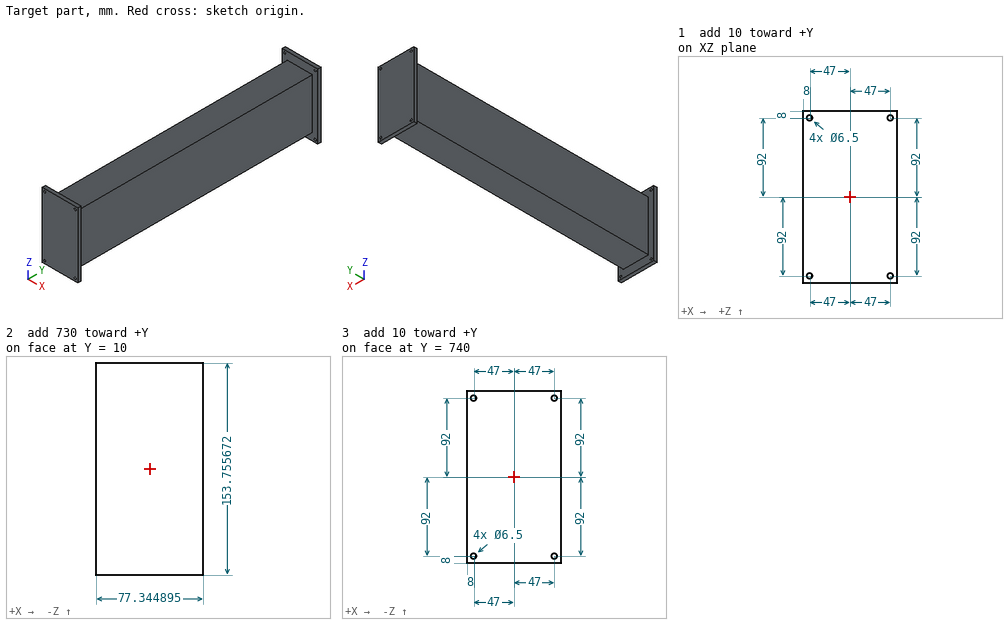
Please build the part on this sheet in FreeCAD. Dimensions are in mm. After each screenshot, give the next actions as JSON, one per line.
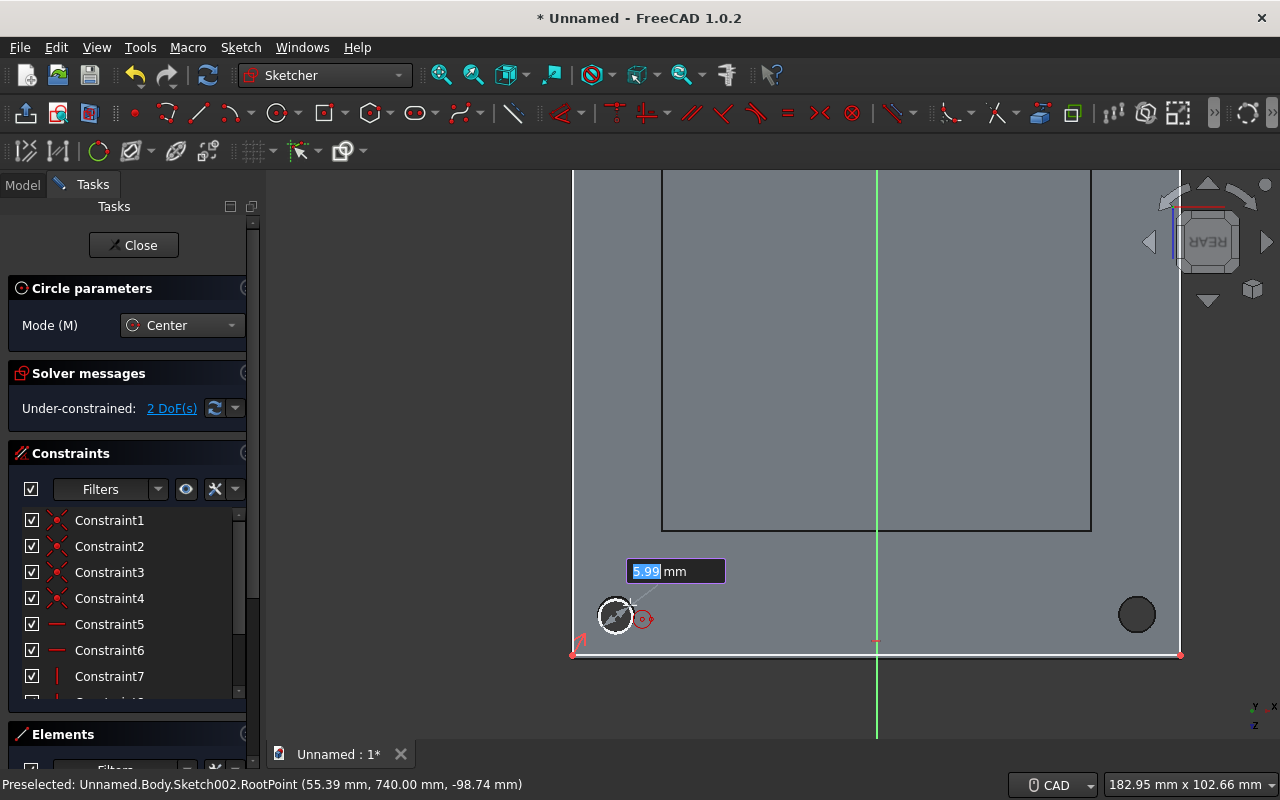
{"action": "left_click", "coordinate": [629, 602]}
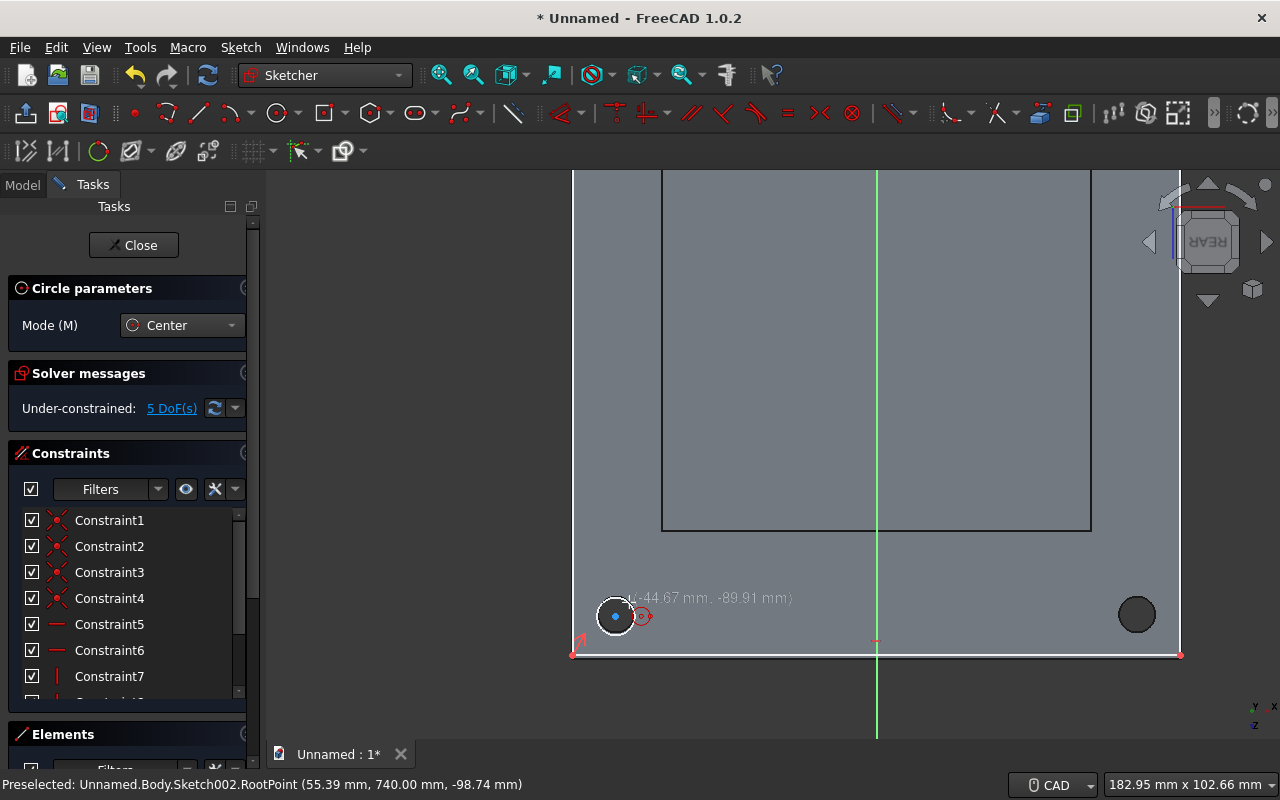
{"action": "scroll", "coordinate": [630, 605], "scroll_direction": "down", "scroll_amount": 6}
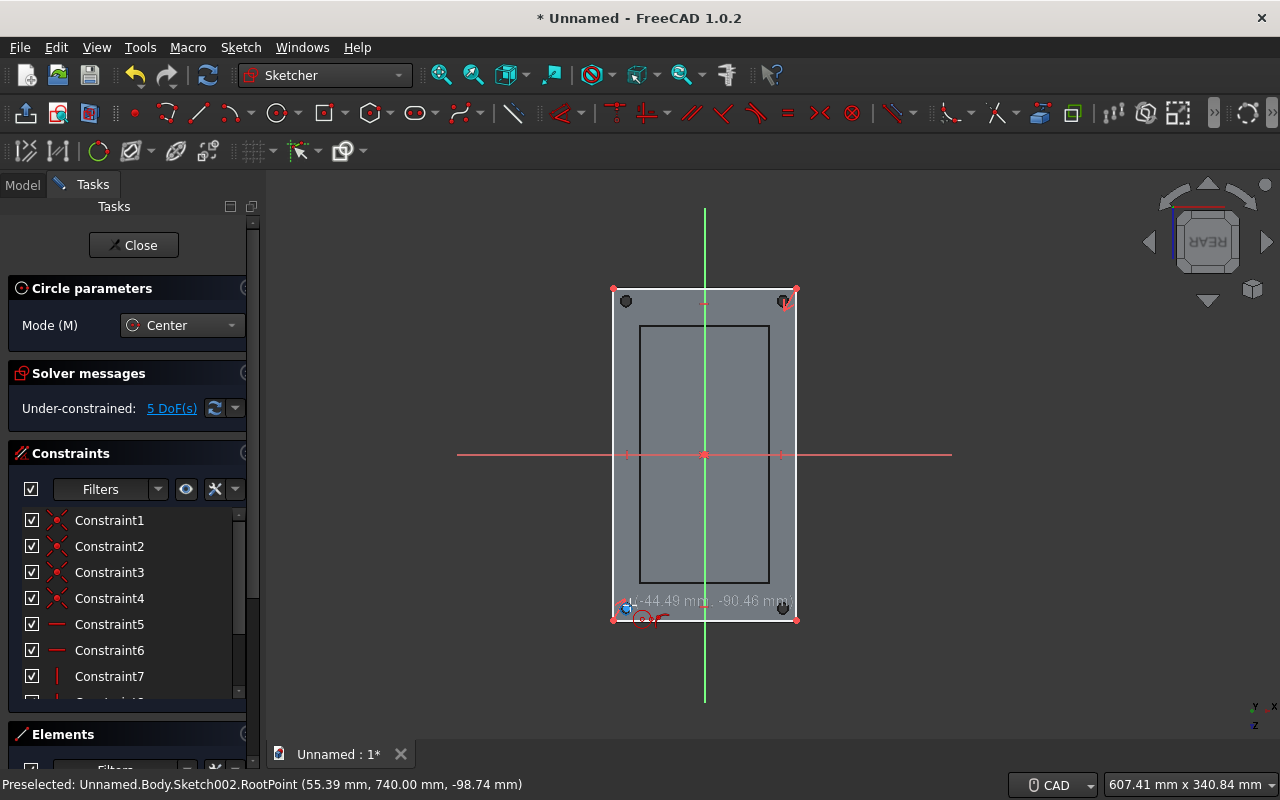
{"action": "scroll", "coordinate": [783, 608], "scroll_direction": "up", "scroll_amount": 8}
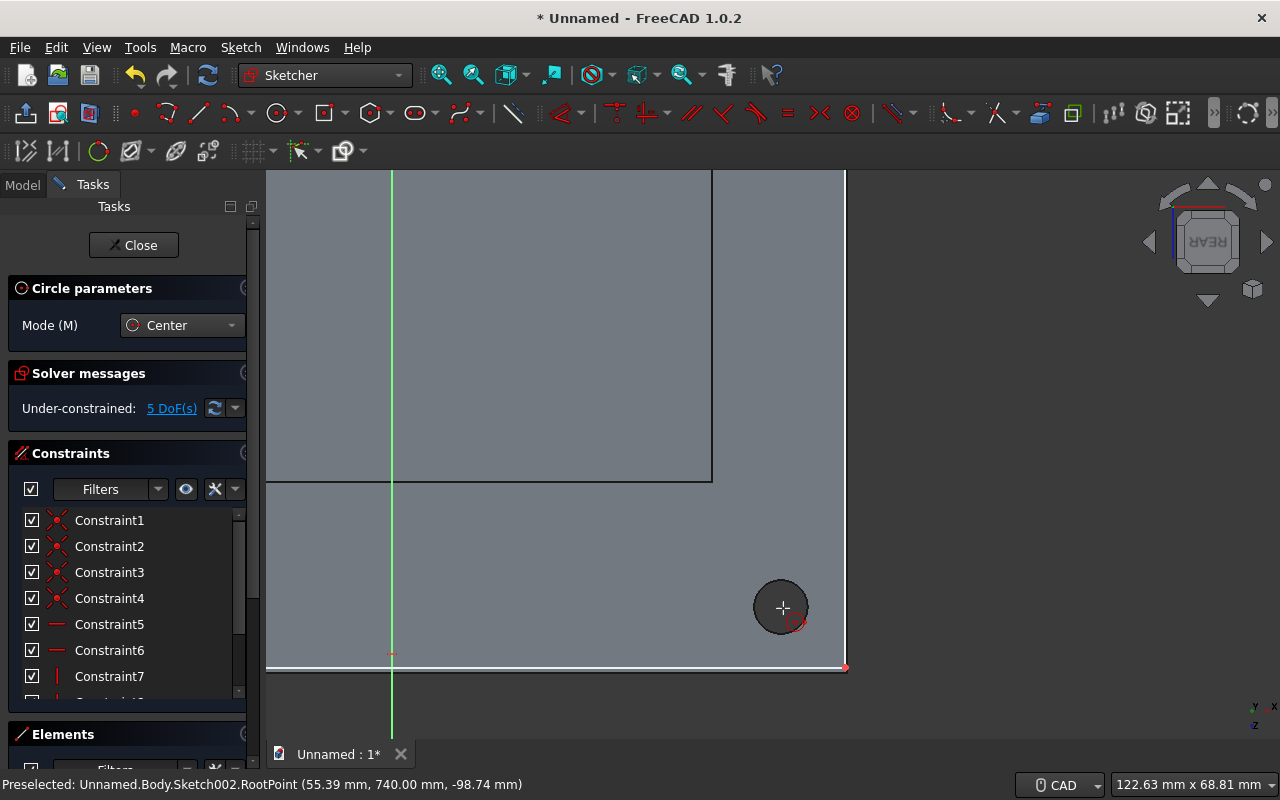
{"action": "scroll", "coordinate": [783, 608], "scroll_direction": "down", "scroll_amount": 8}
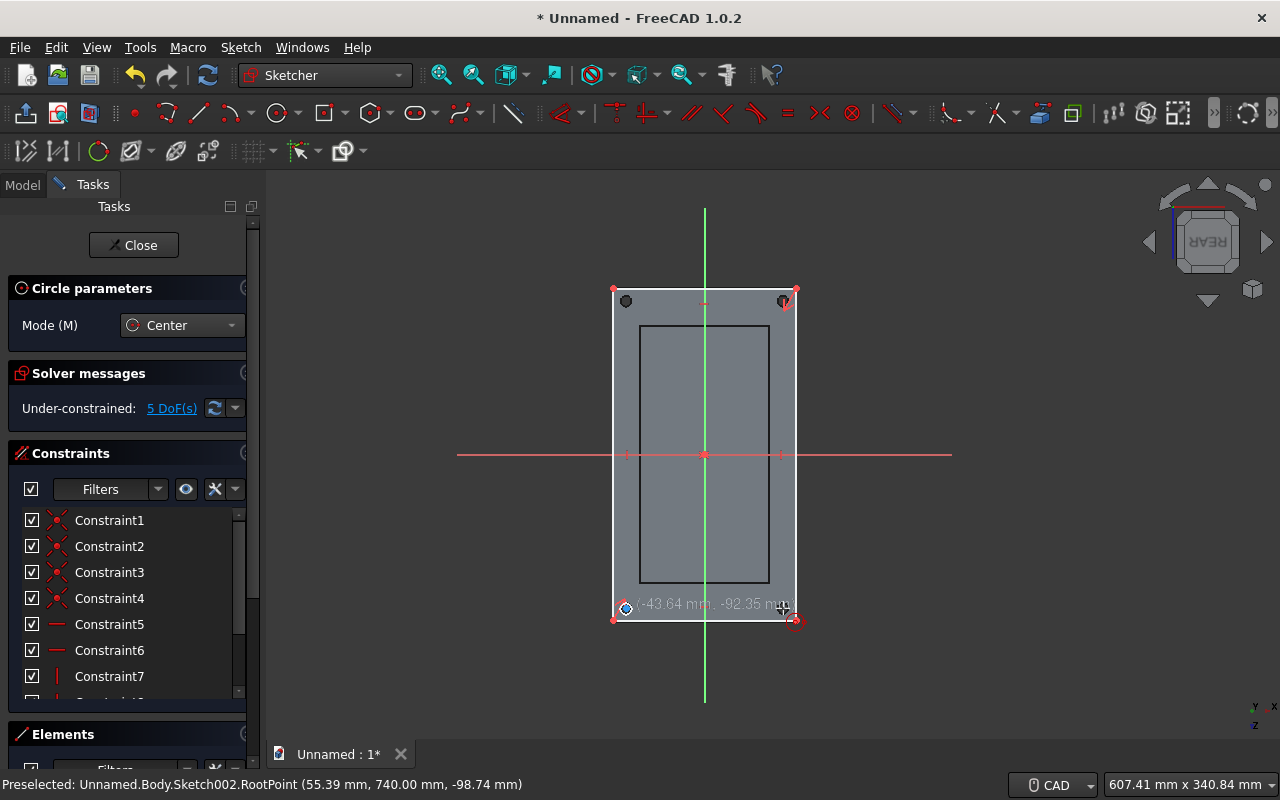
{"action": "left_click", "coordinate": [783, 608]}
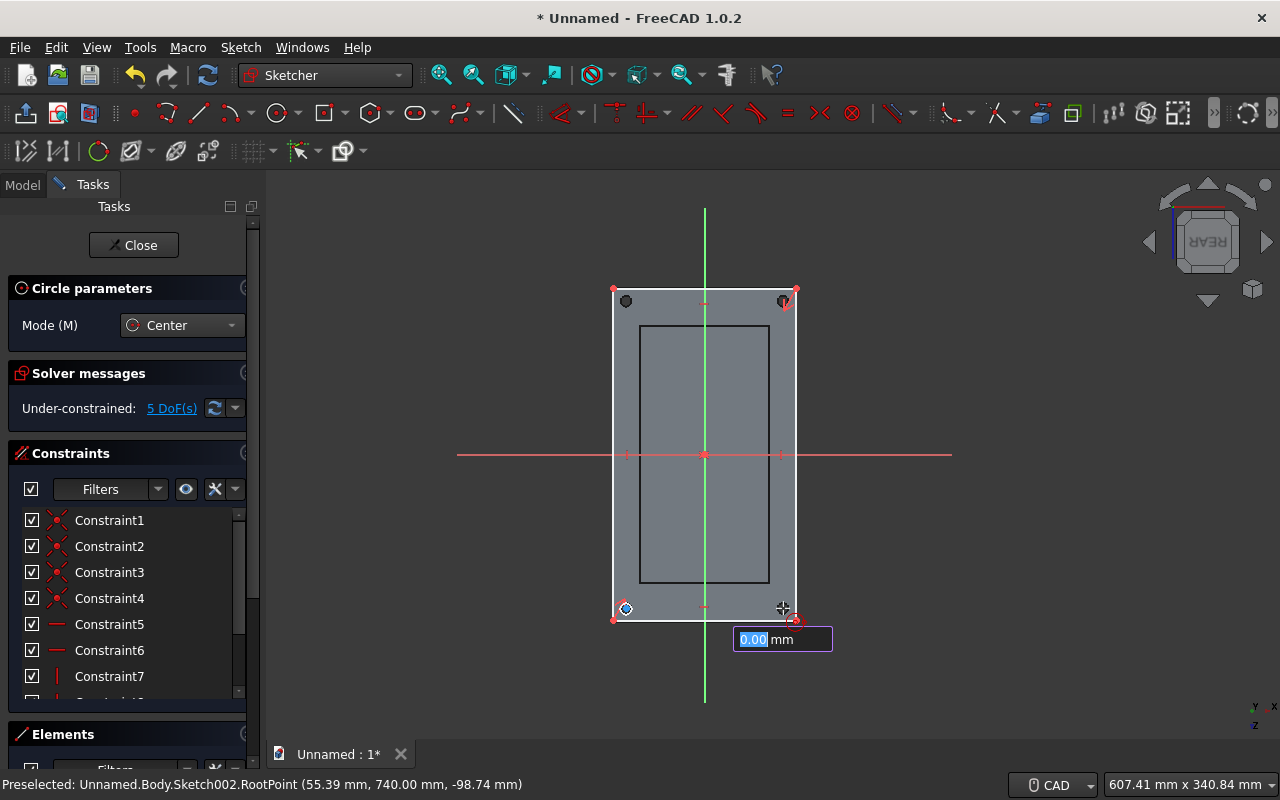
{"action": "scroll", "coordinate": [779, 605], "scroll_direction": "up", "scroll_amount": 6}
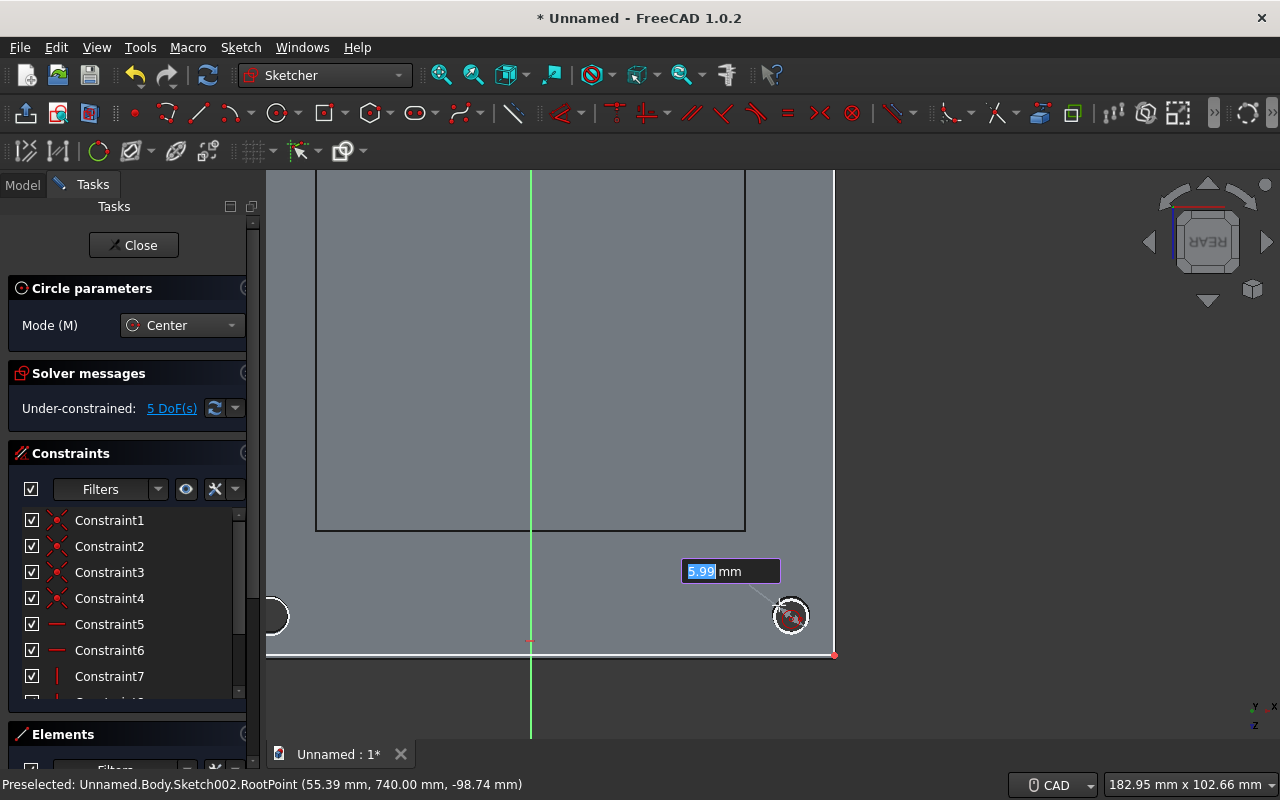
{"action": "left_click", "coordinate": [778, 602]}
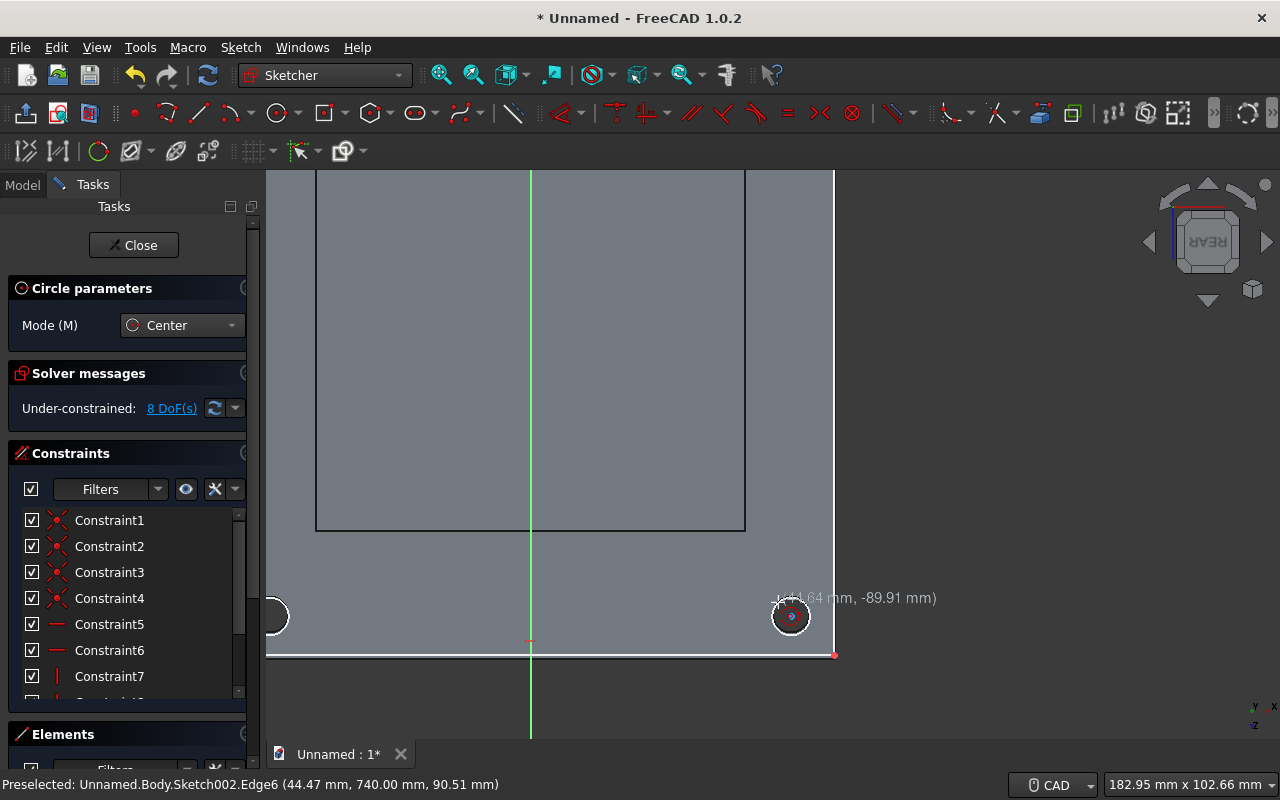
{"action": "scroll", "coordinate": [779, 605], "scroll_direction": "down", "scroll_amount": 6}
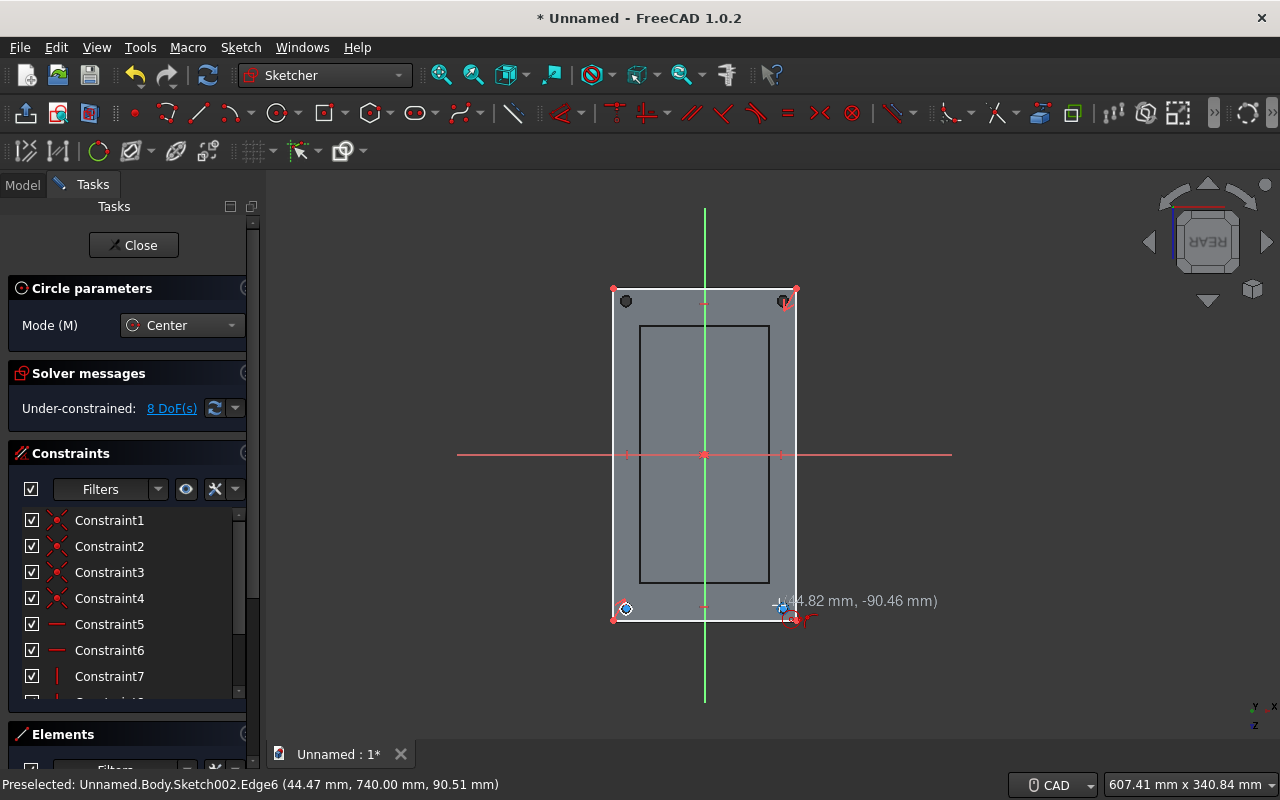
{"action": "scroll", "coordinate": [626, 301], "scroll_direction": "up", "scroll_amount": 8}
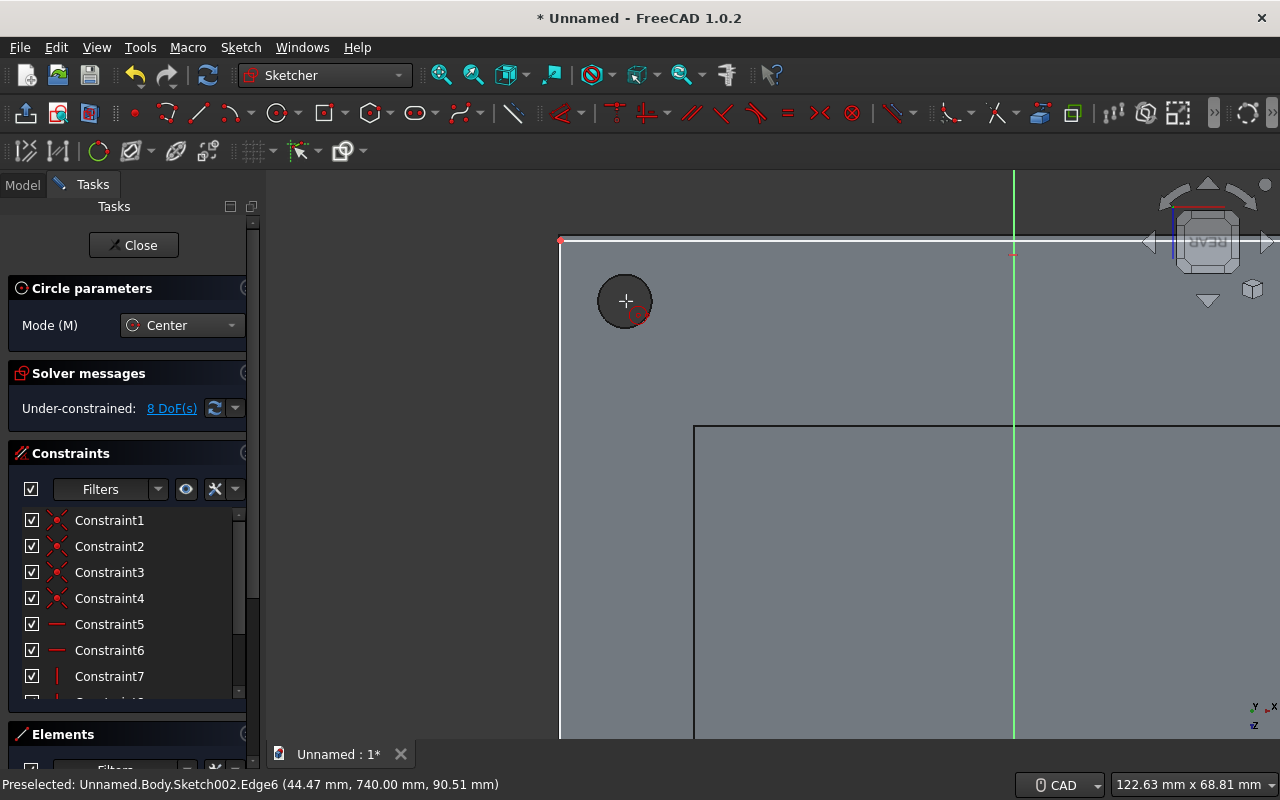
{"action": "scroll", "coordinate": [626, 301], "scroll_direction": "down", "scroll_amount": 8}